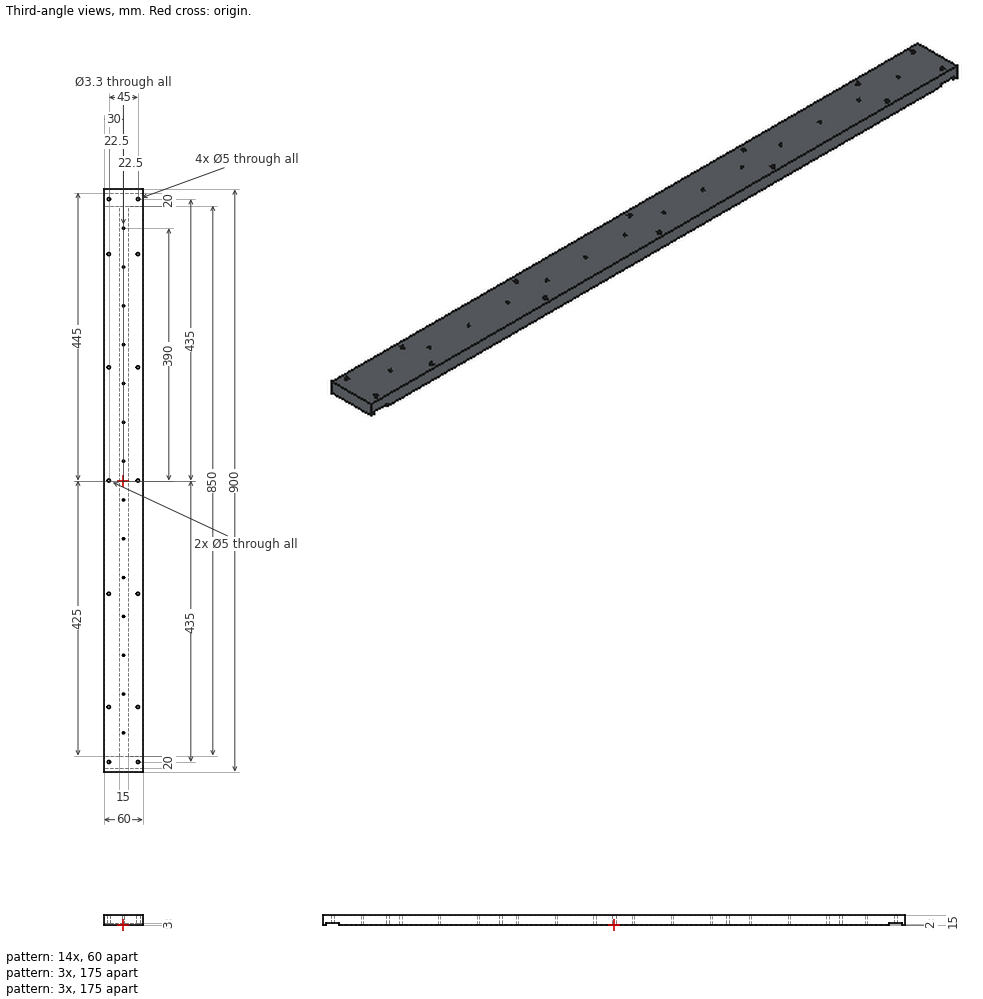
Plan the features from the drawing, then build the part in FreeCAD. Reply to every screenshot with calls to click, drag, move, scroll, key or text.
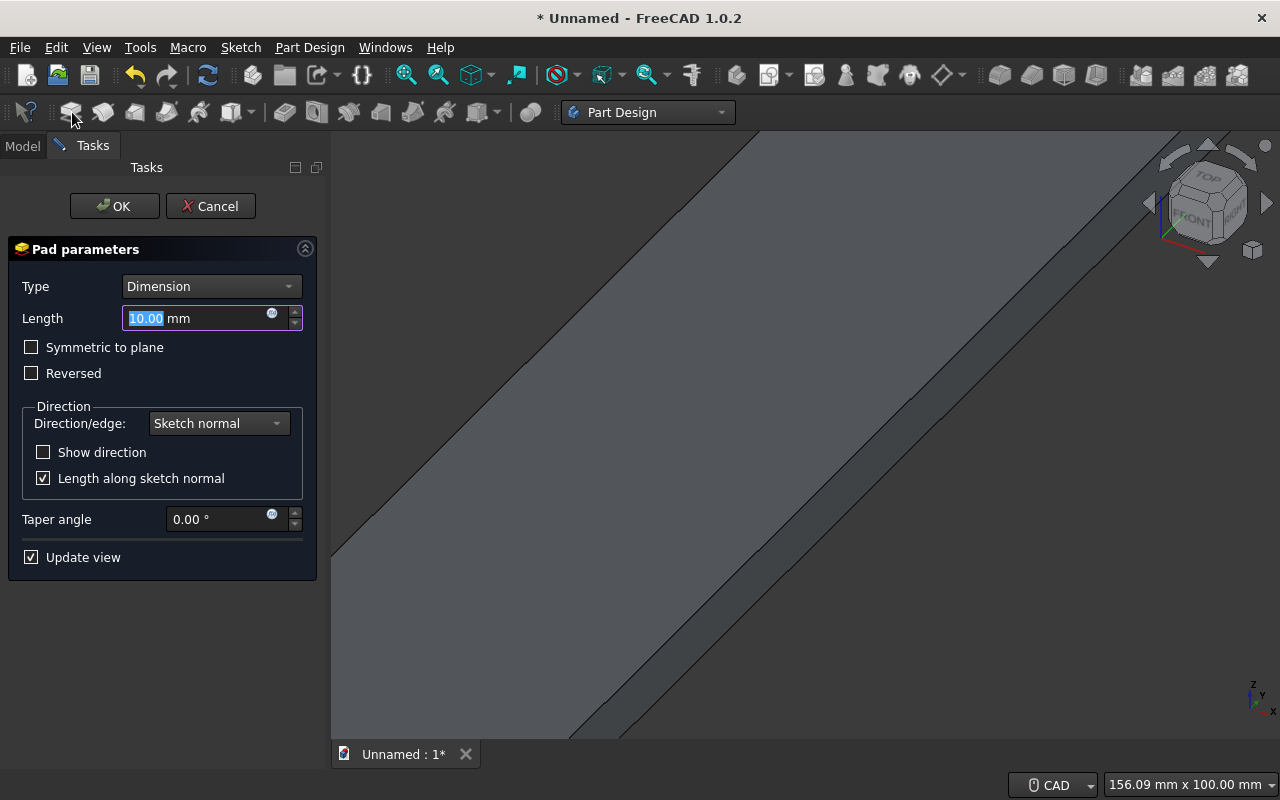
text(15)
key(Tab)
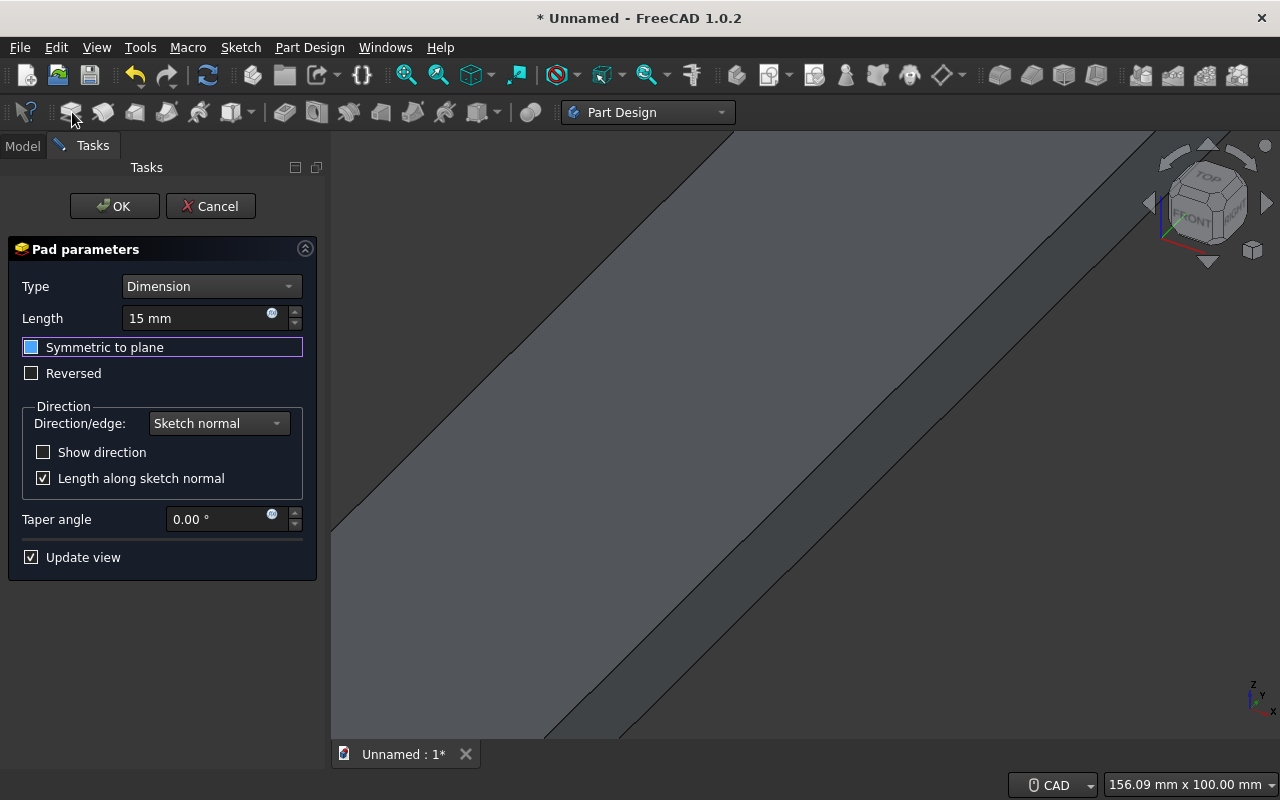
click(115, 206)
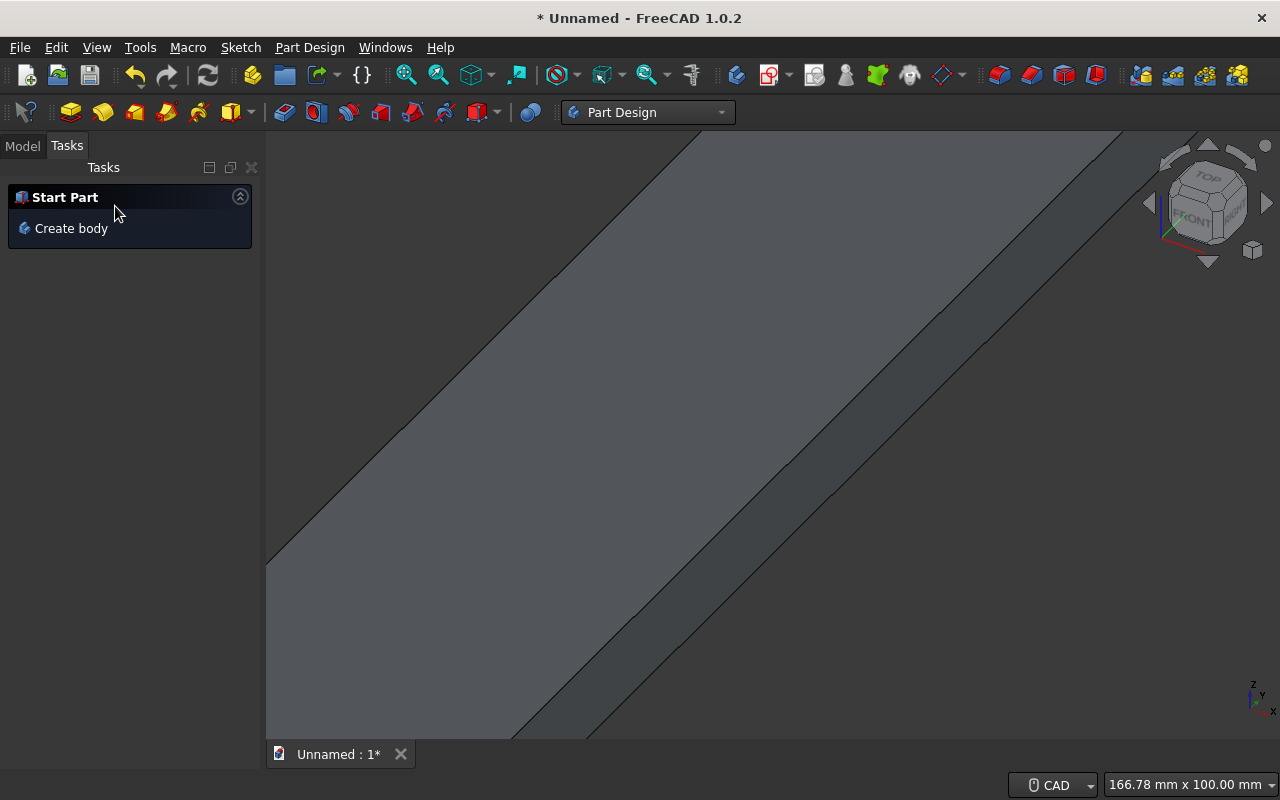
key(v)
key(f)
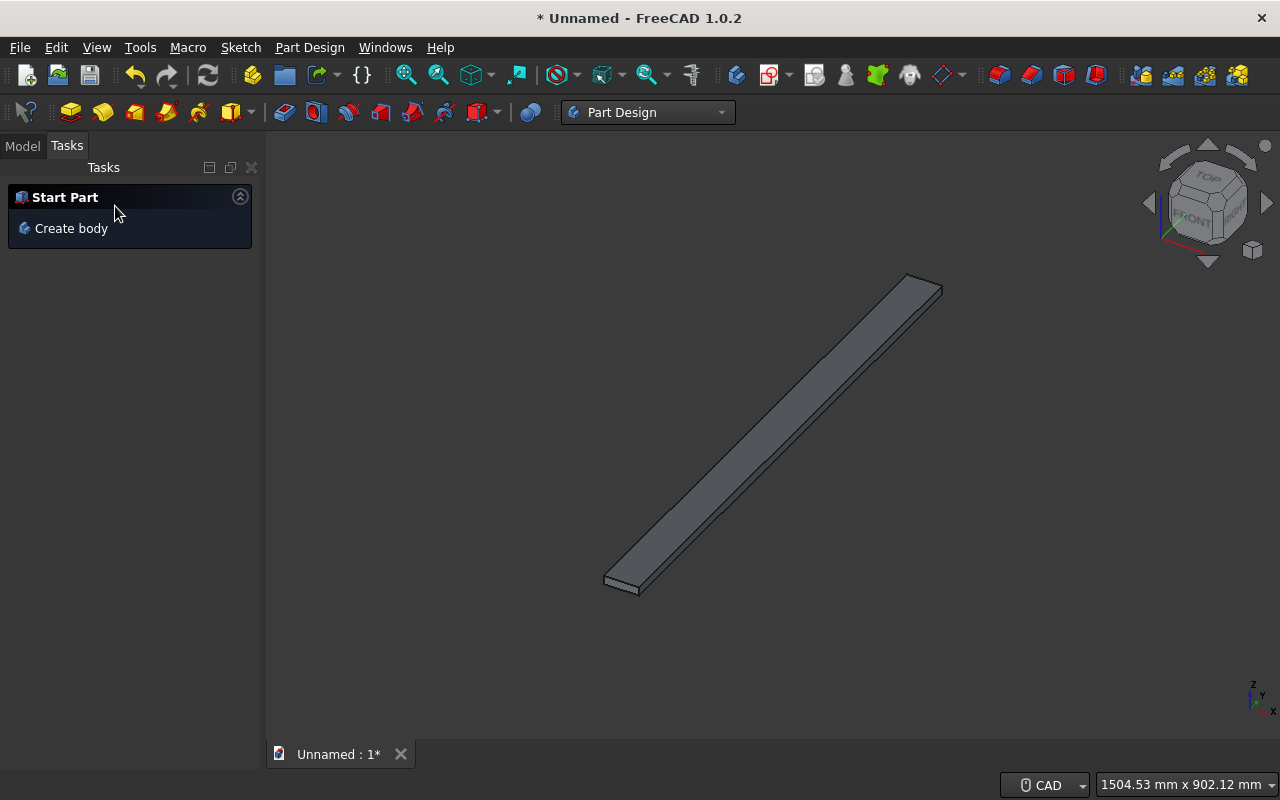
click(770, 76)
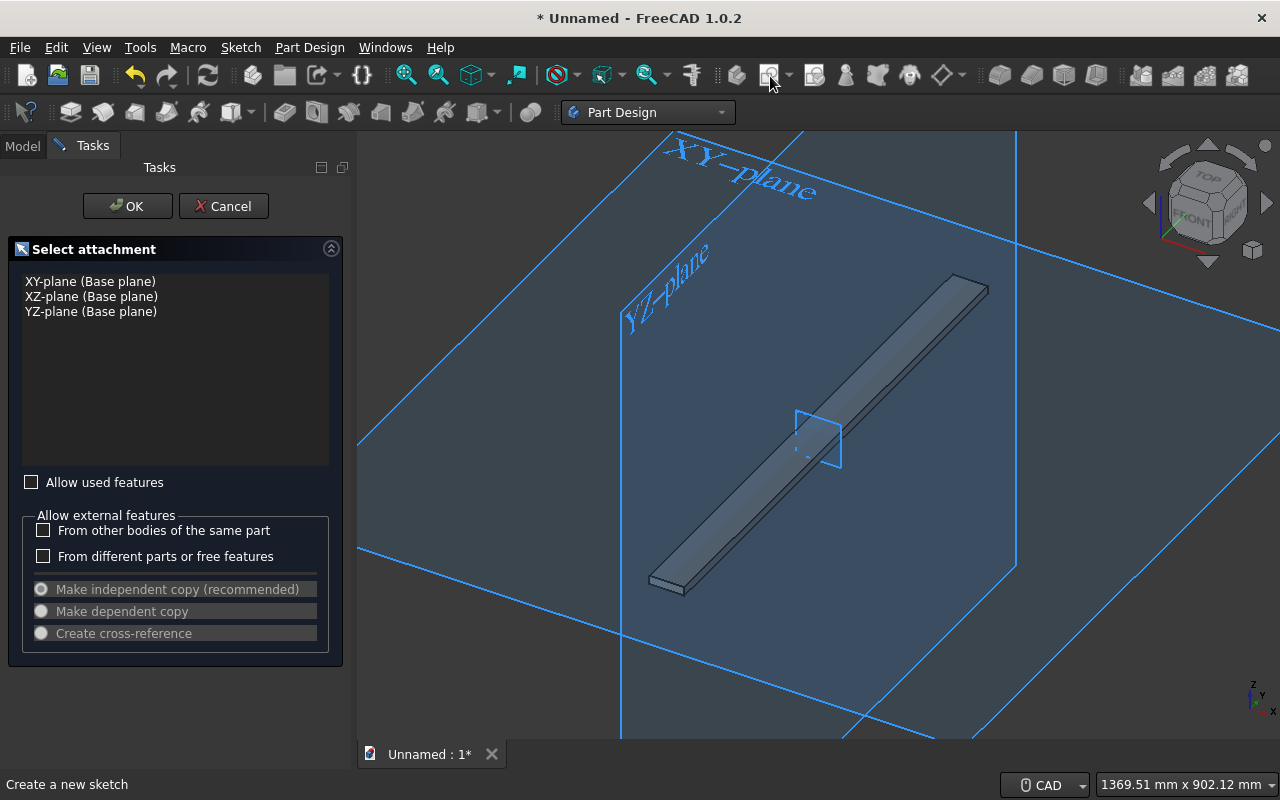
click(82, 282)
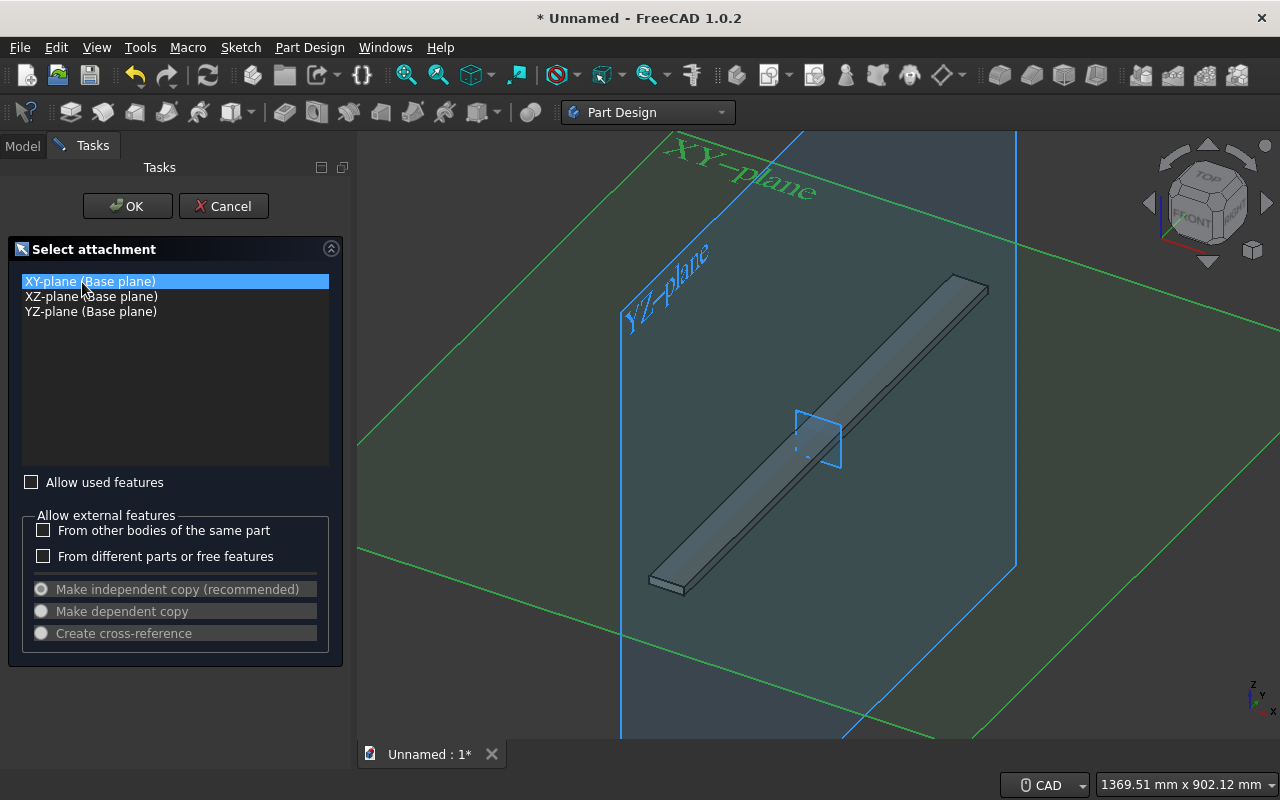
click(128, 206)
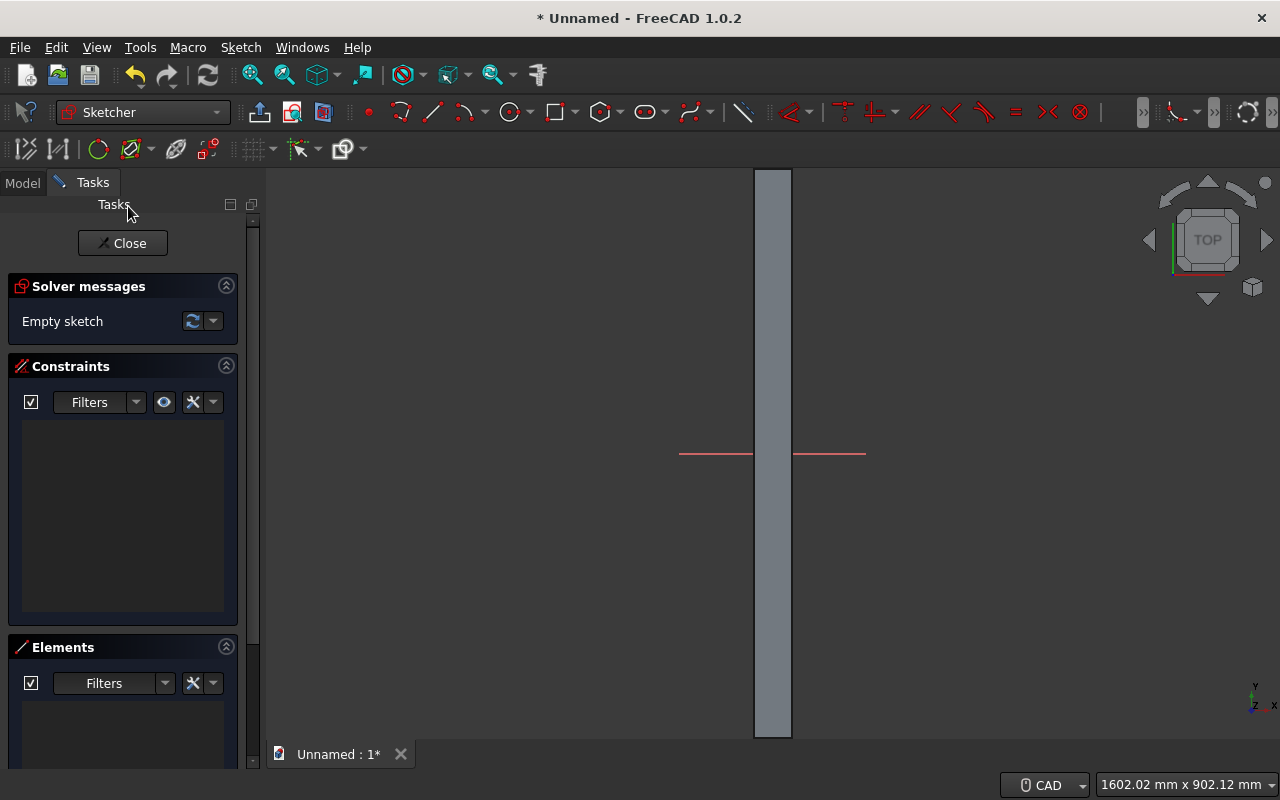
key(q)
key(s)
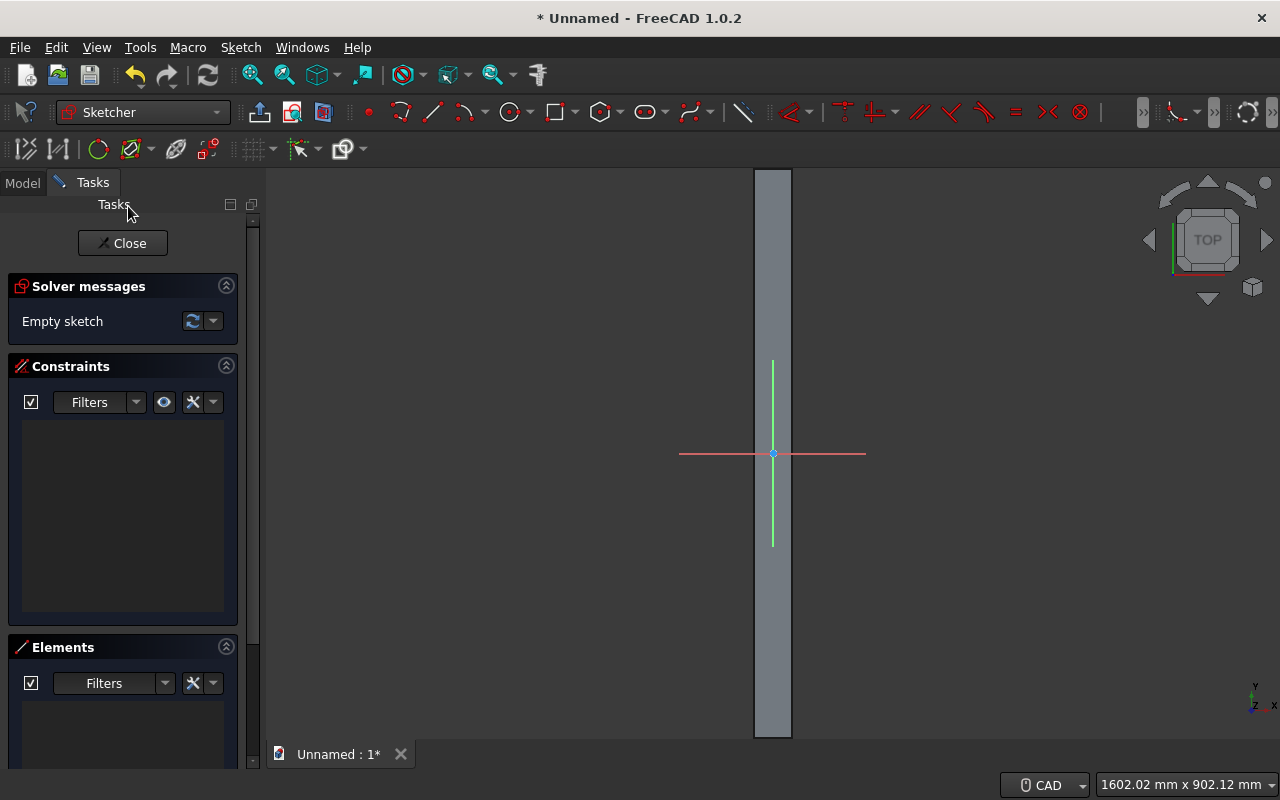
scroll(565, 453, down, 2)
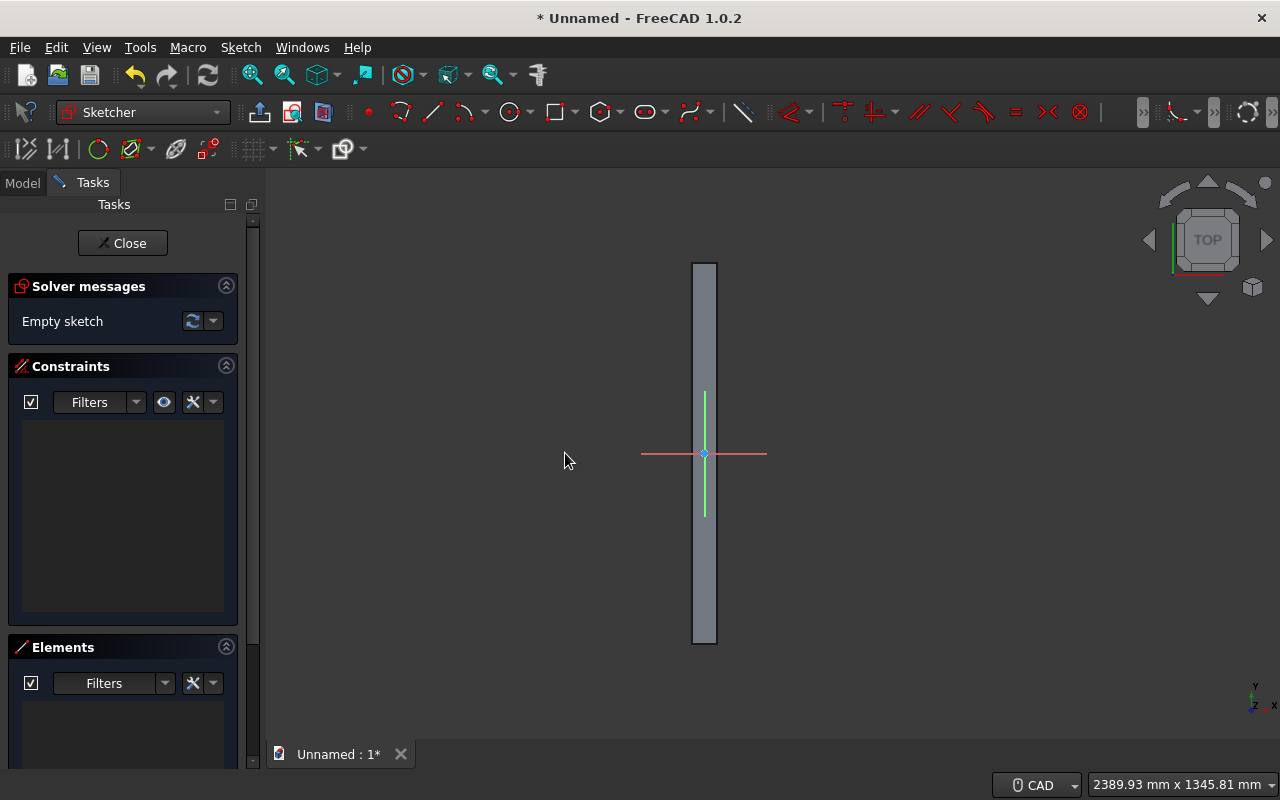
key(g)
key(r)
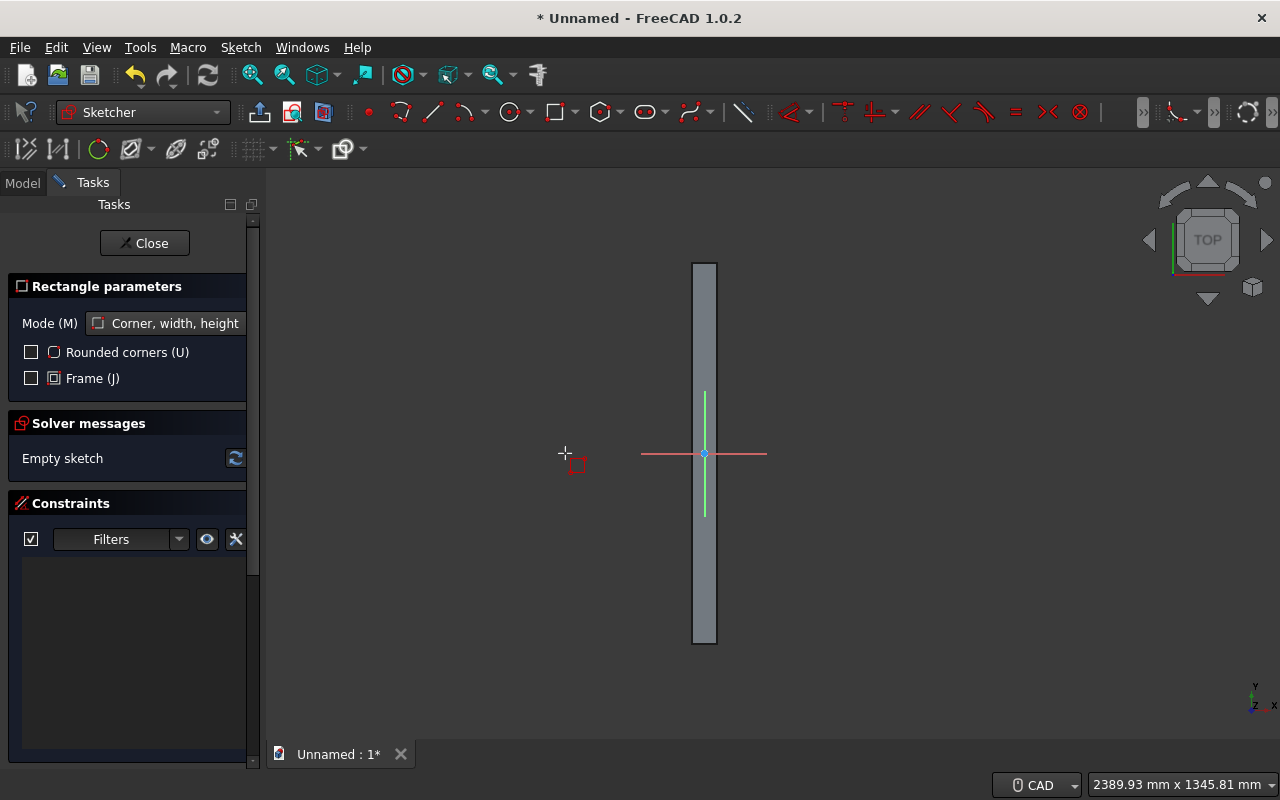
scroll(692, 265, up, 4)